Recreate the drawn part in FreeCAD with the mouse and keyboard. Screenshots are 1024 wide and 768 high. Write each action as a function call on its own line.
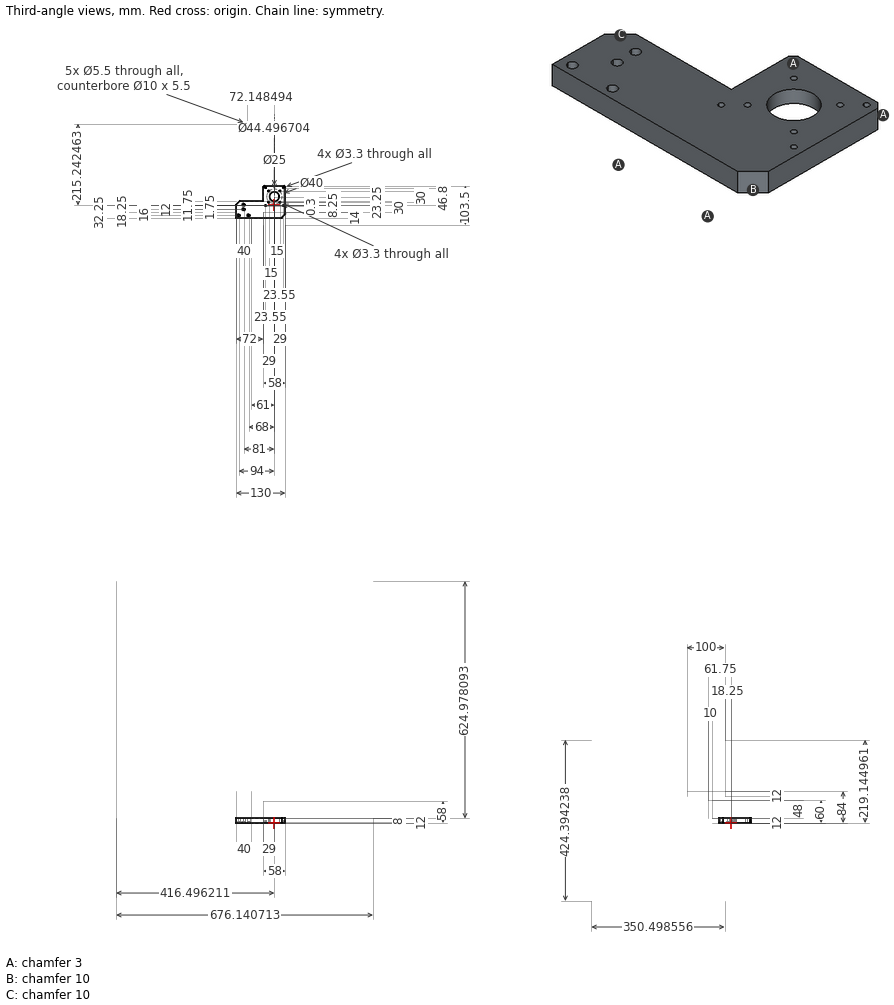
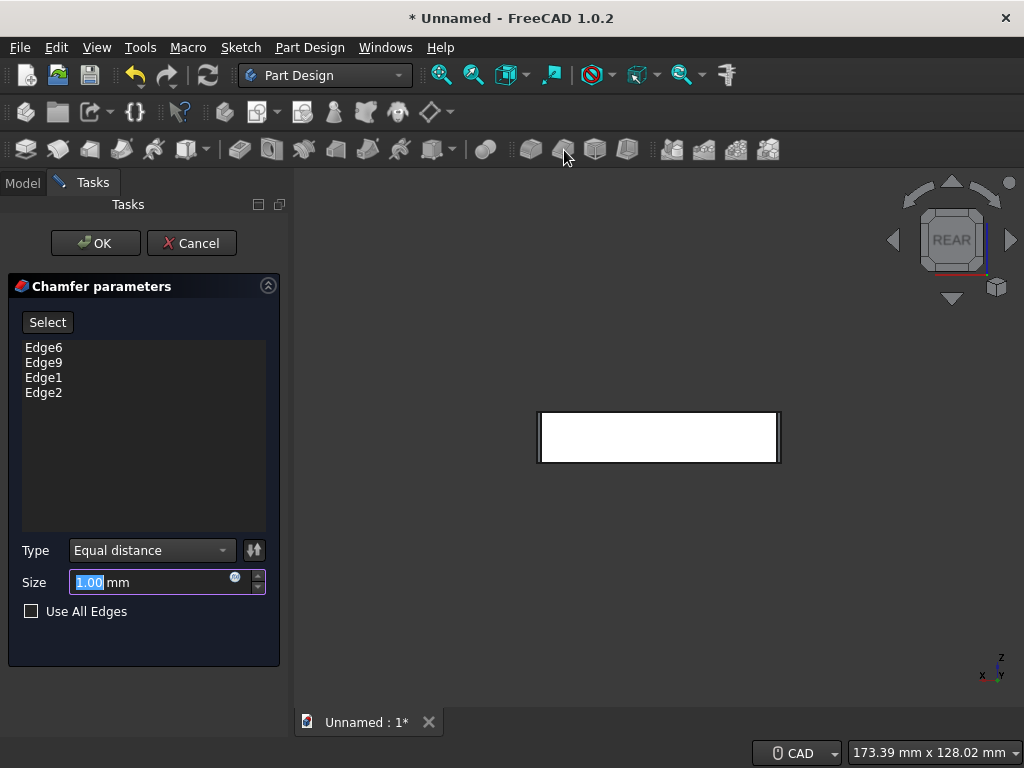
text(3)
key(Tab)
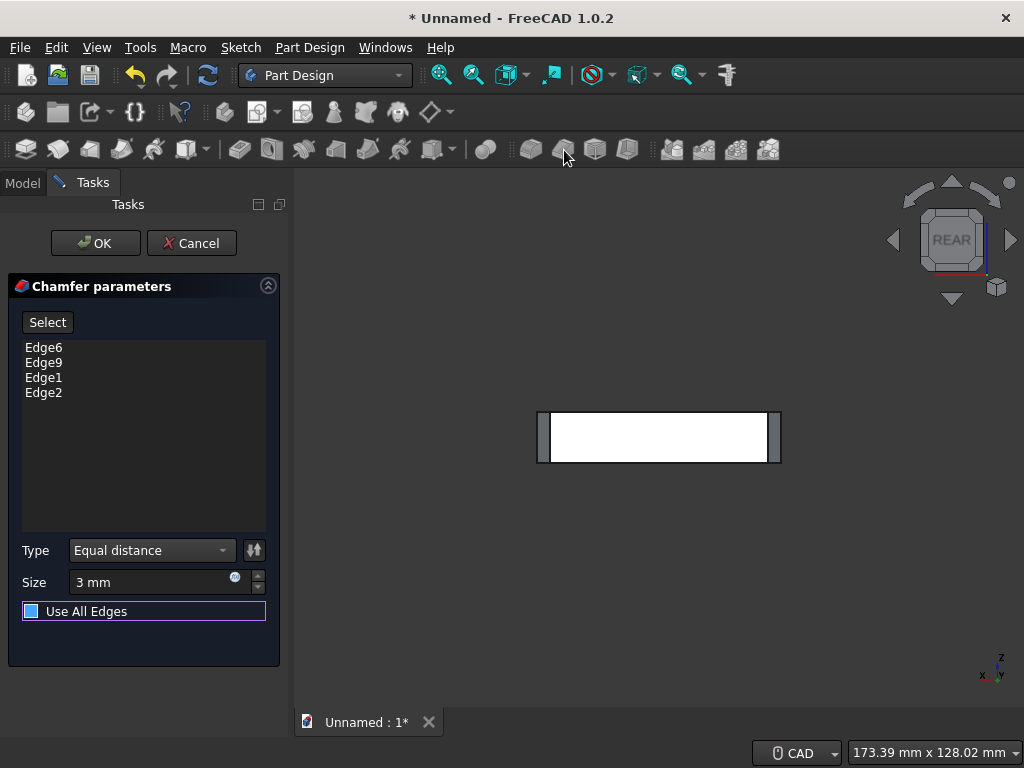
click(96, 243)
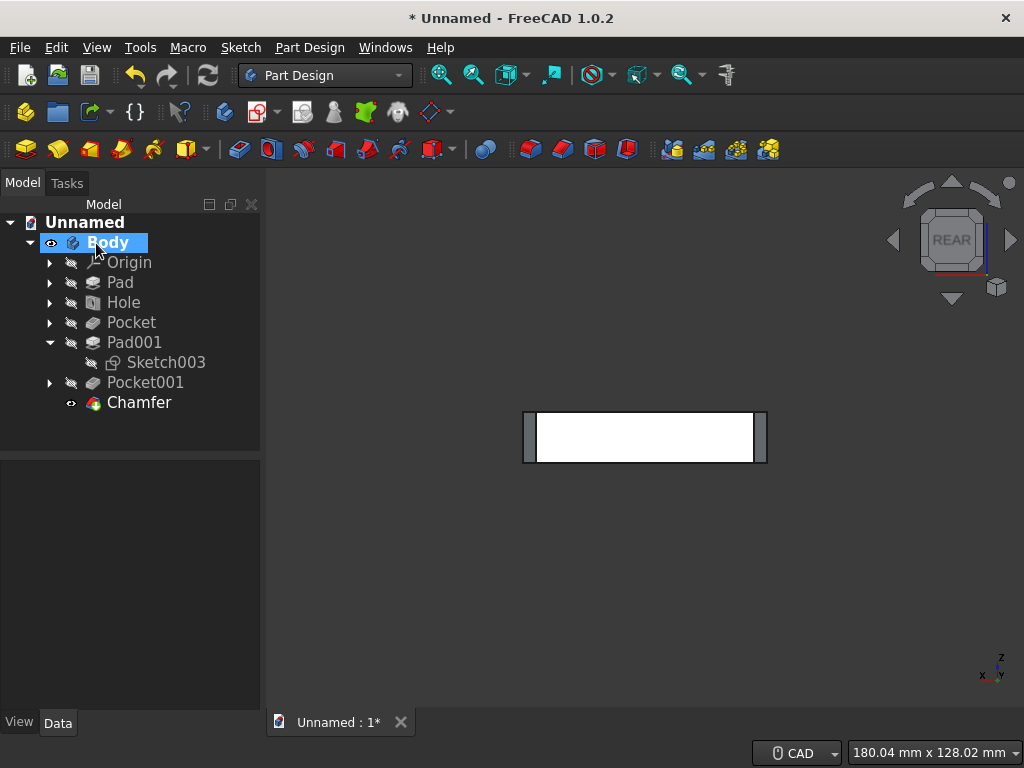
click(442, 76)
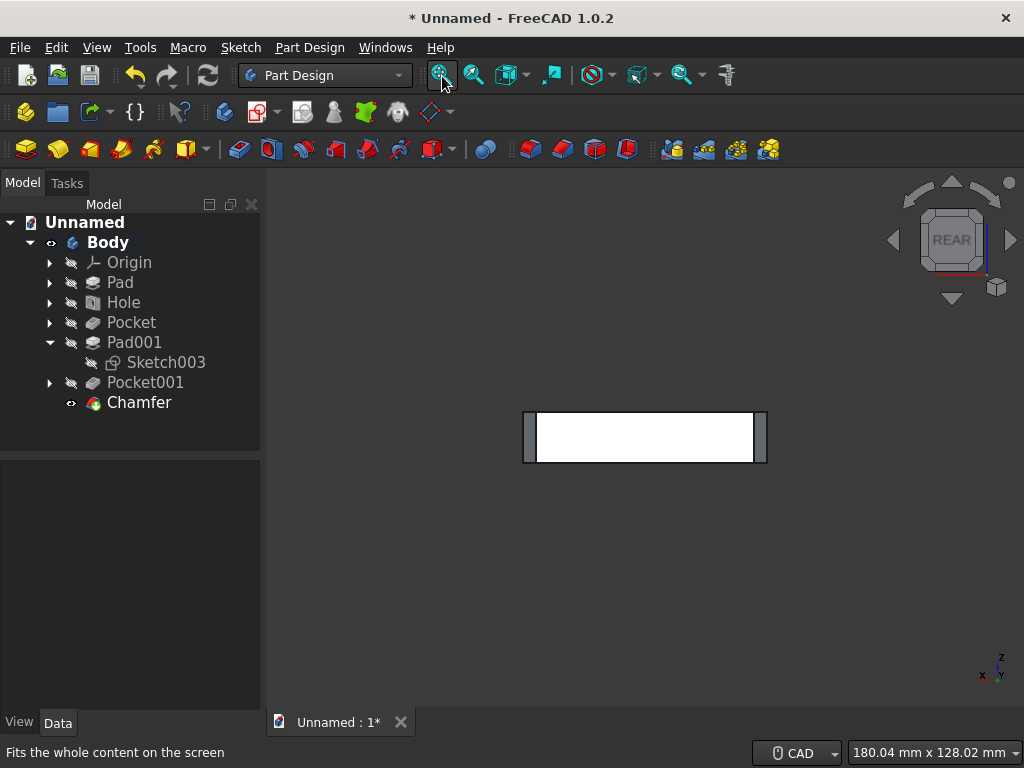
key(6)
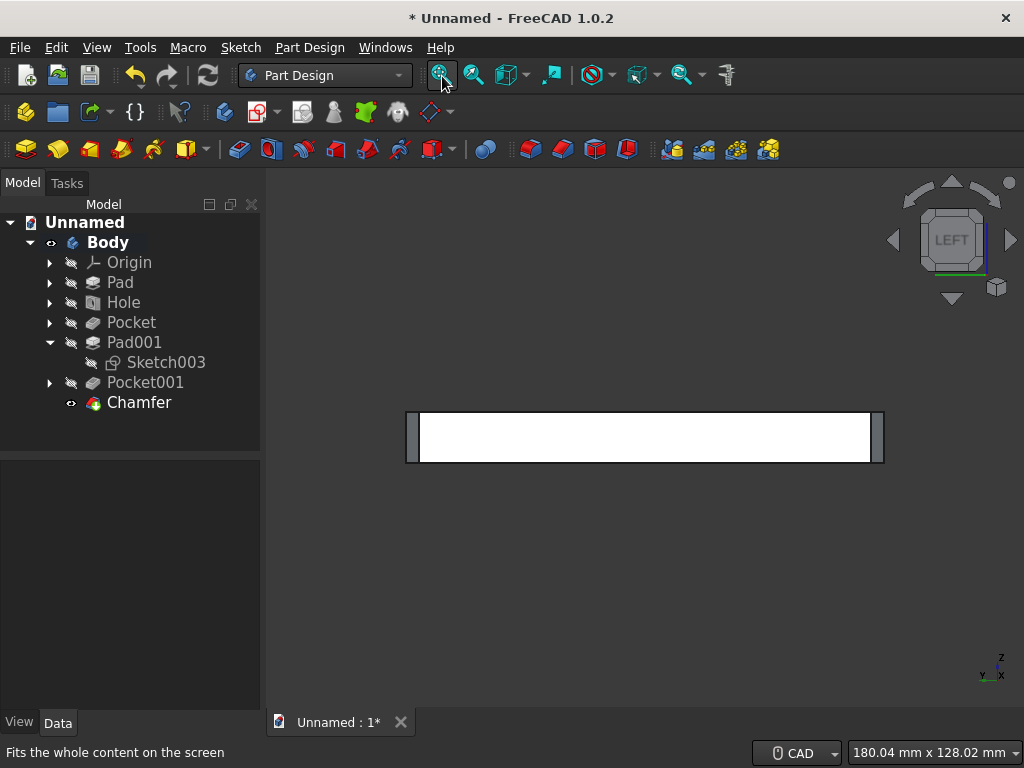
click(451, 436)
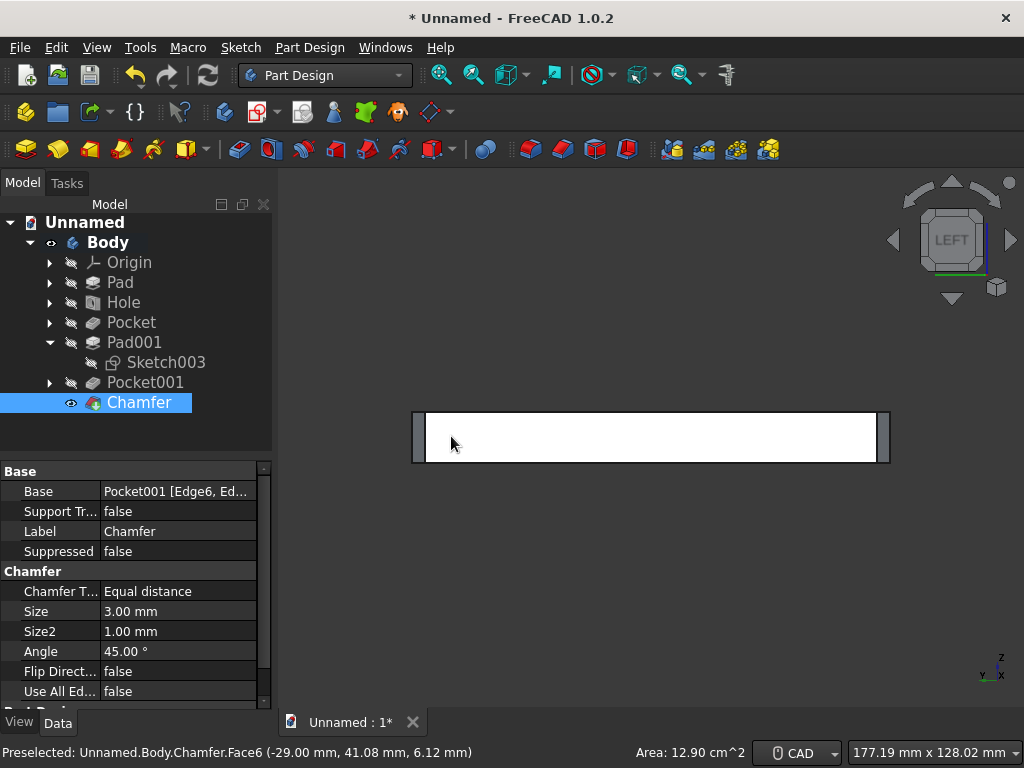
click(258, 112)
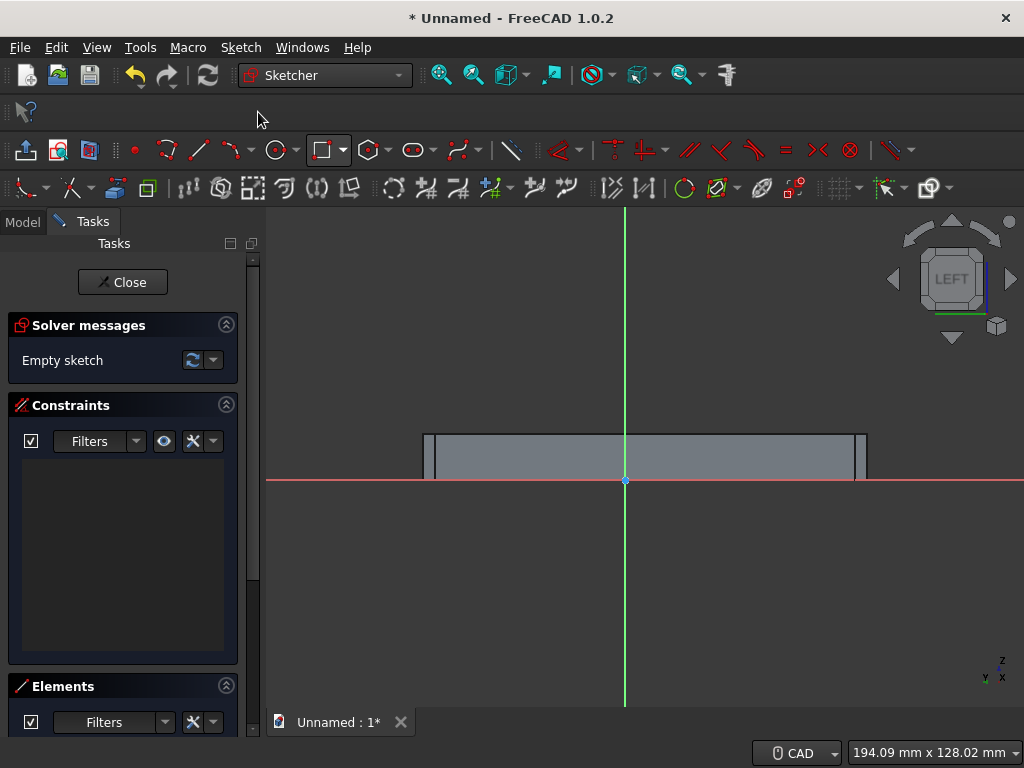
scroll(382, 458, down, 8)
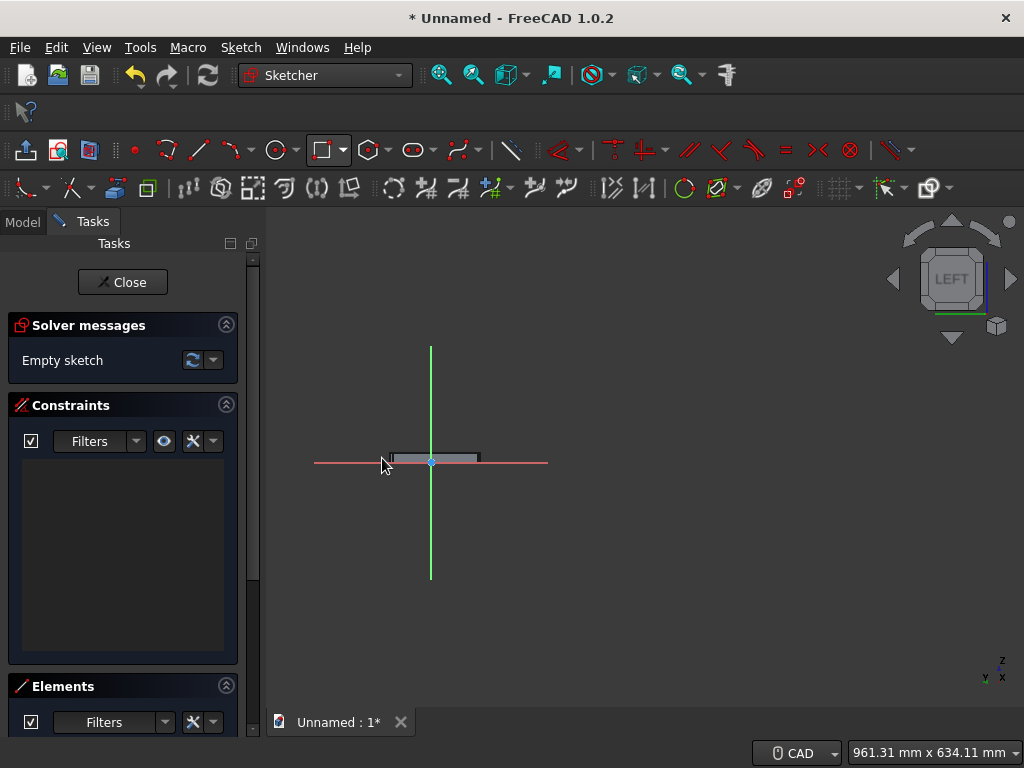
key(g)
key(r)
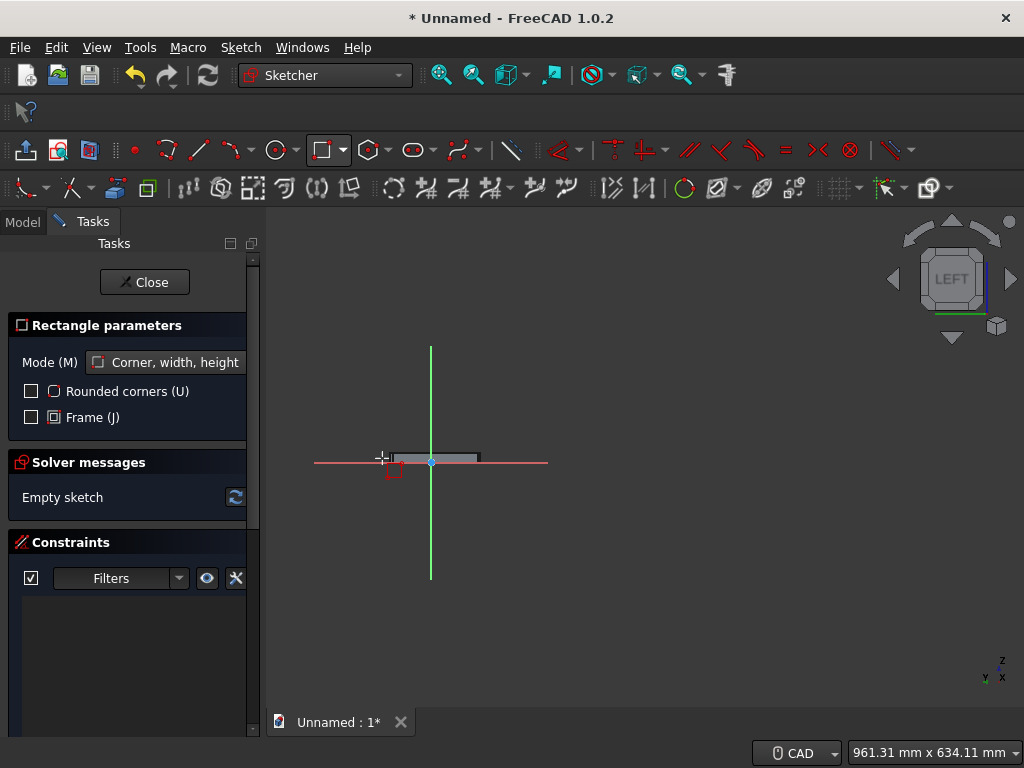
click(446, 290)
move(722, 625)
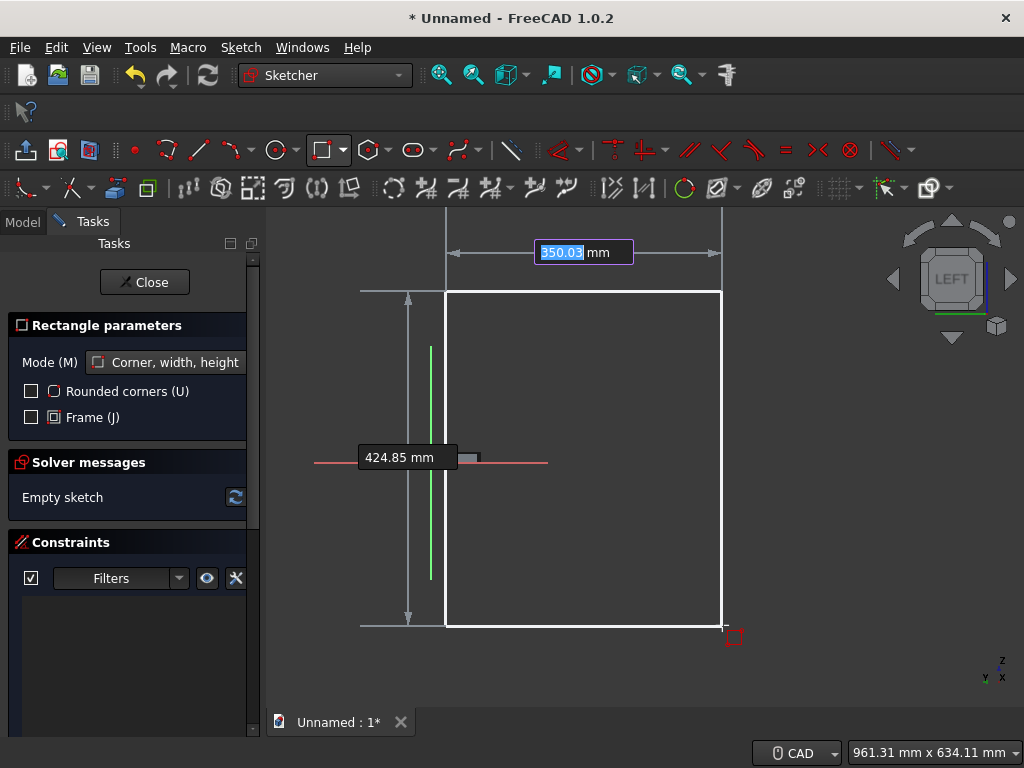
text(350.498556)
key(Tab)
text(424.394238)
key(Return)
key(Escape)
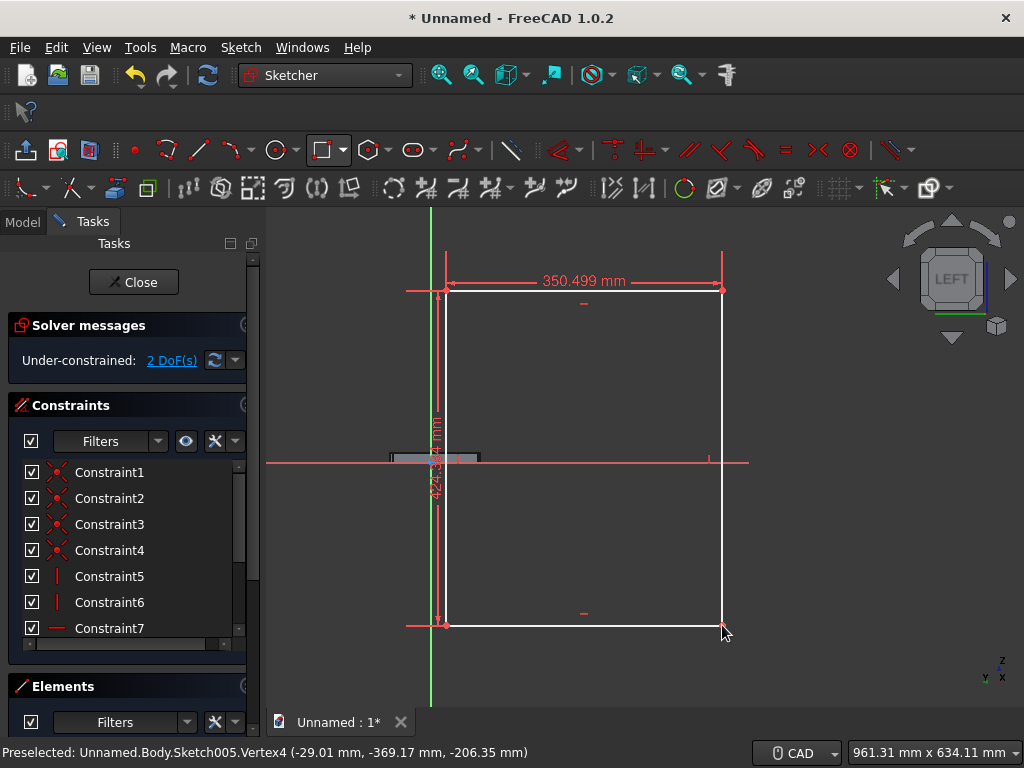
key(d)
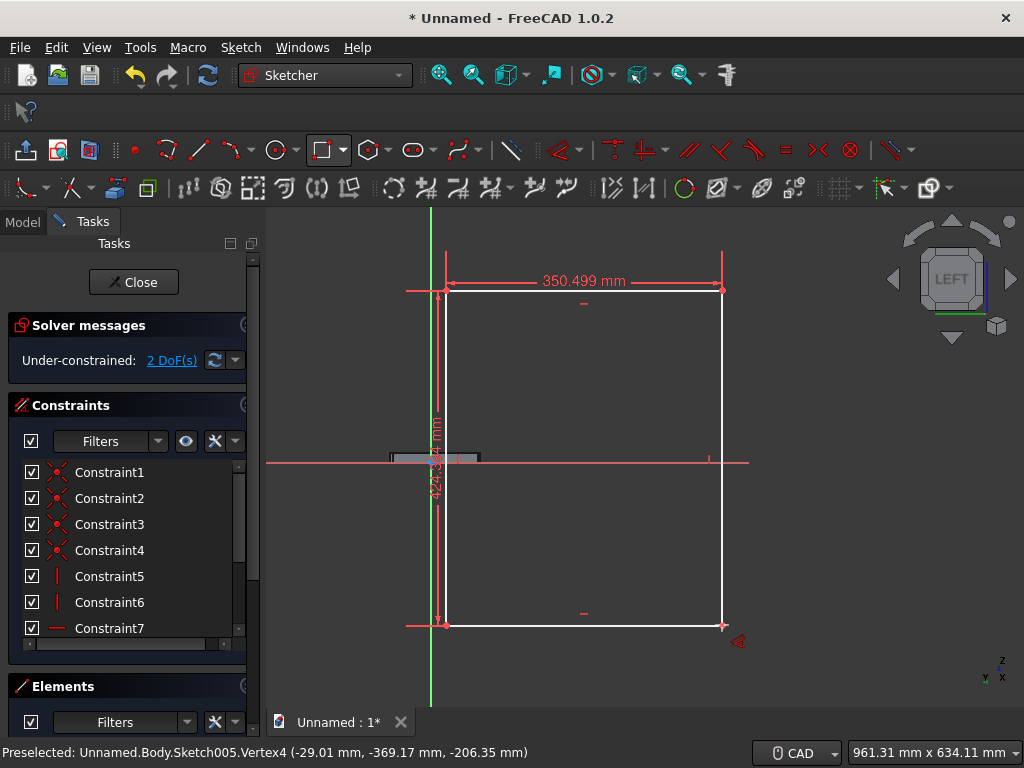
scroll(446, 291, up, 6)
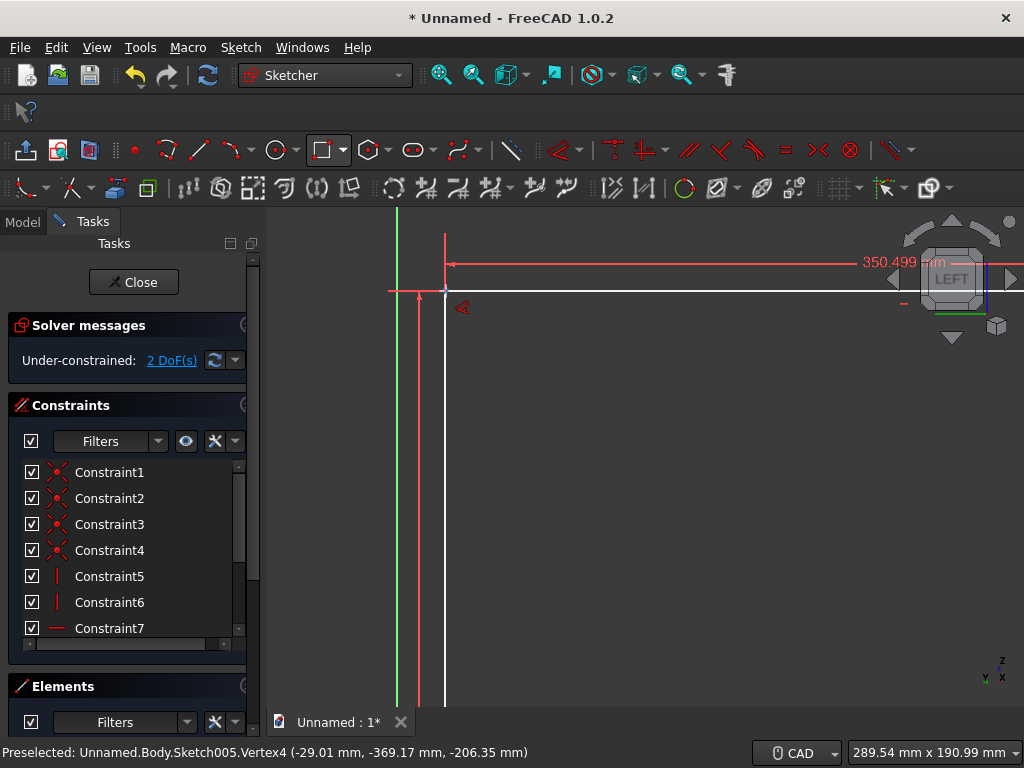
click(445, 291)
click(421, 257)